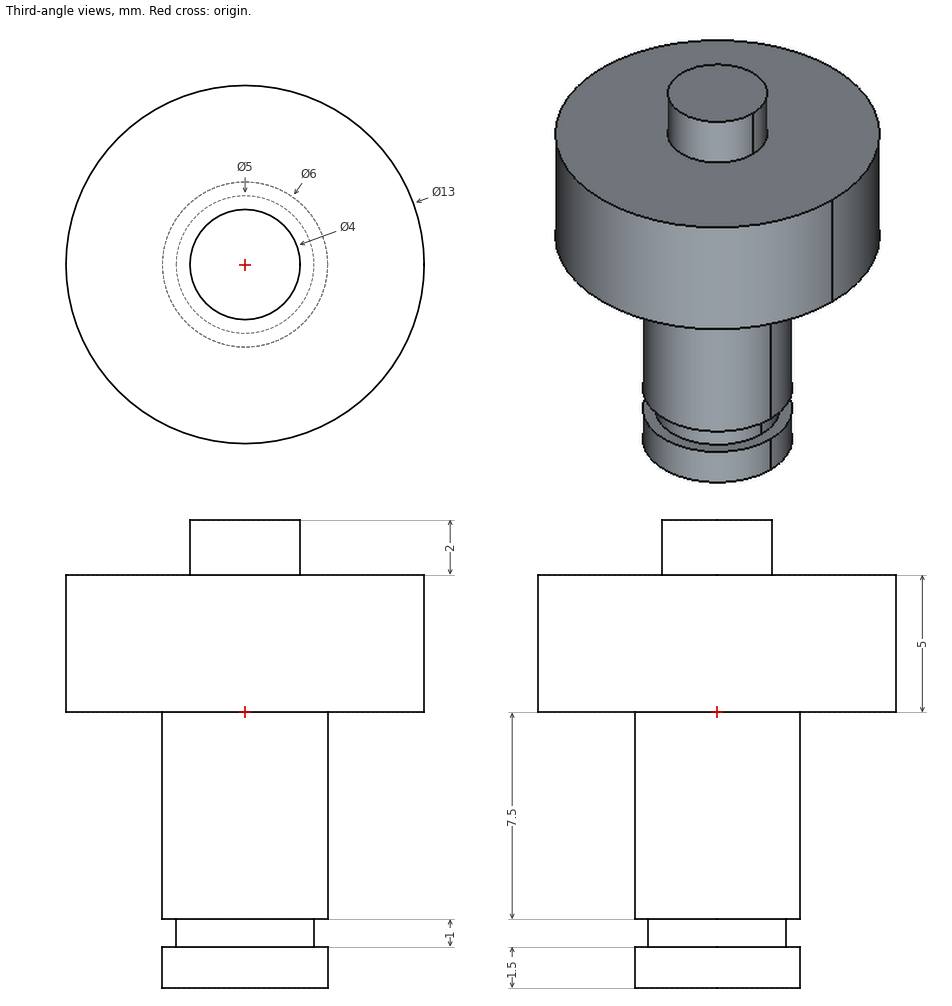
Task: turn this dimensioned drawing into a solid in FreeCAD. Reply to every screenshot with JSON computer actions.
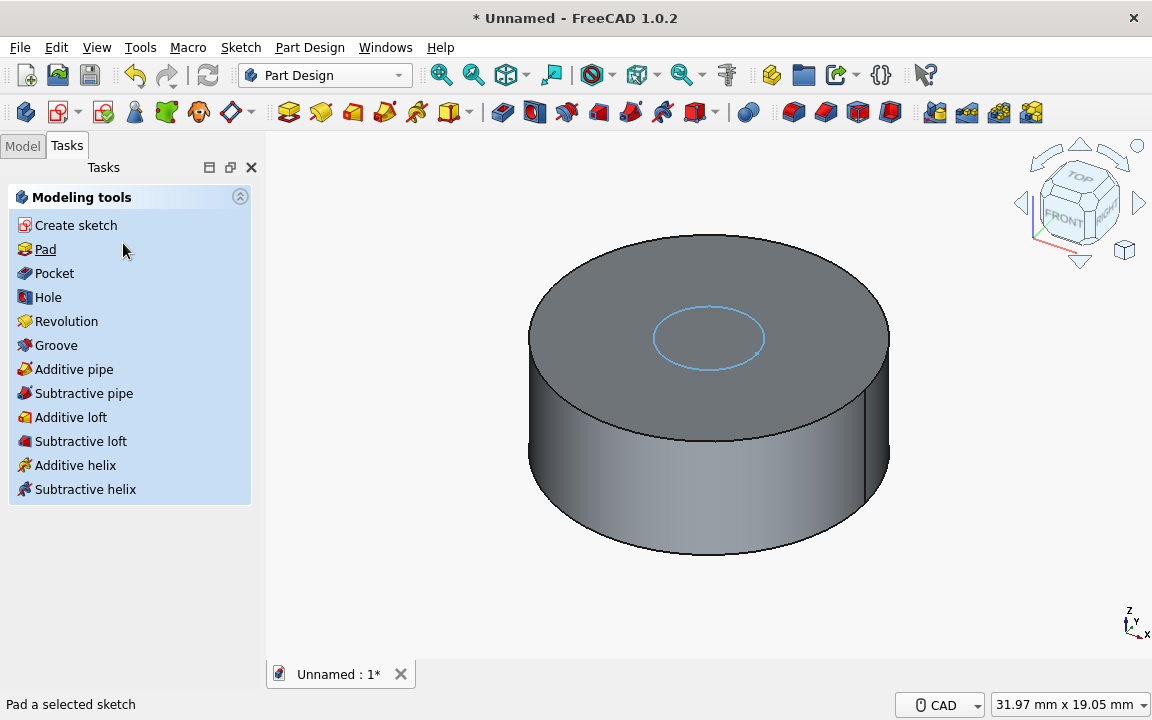
{"action": "left_click", "coordinate": [290, 112]}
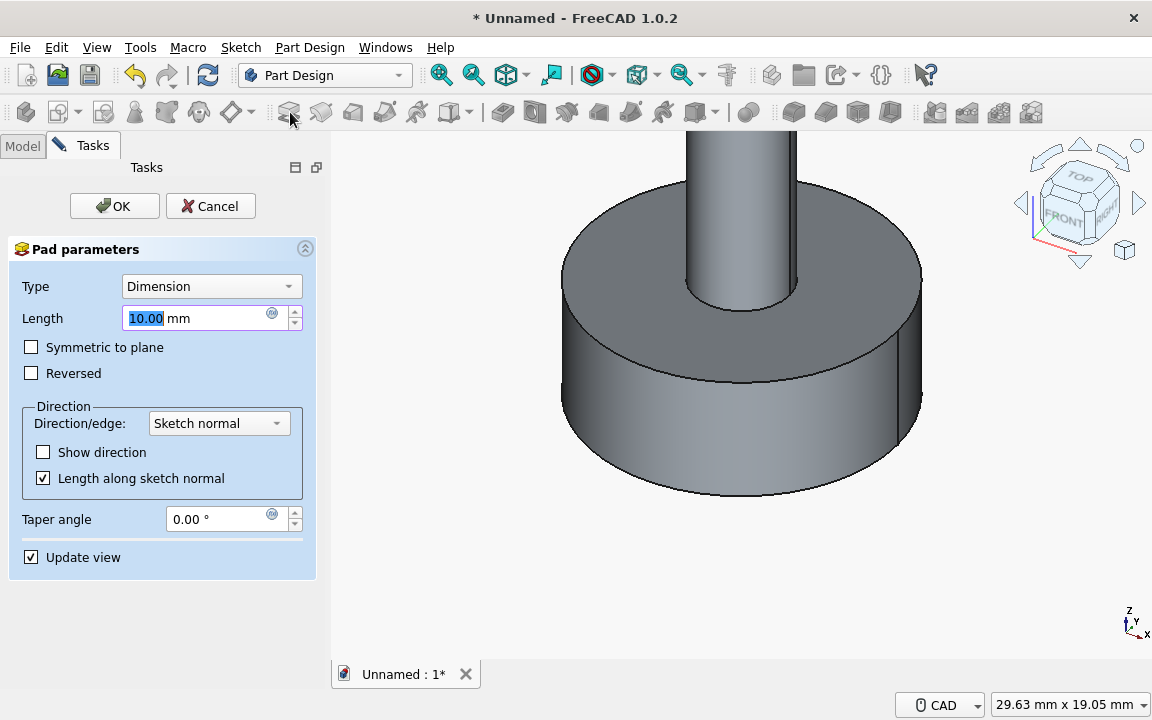
{"action": "type", "text": "2"}
{"action": "key", "text": "Tab"}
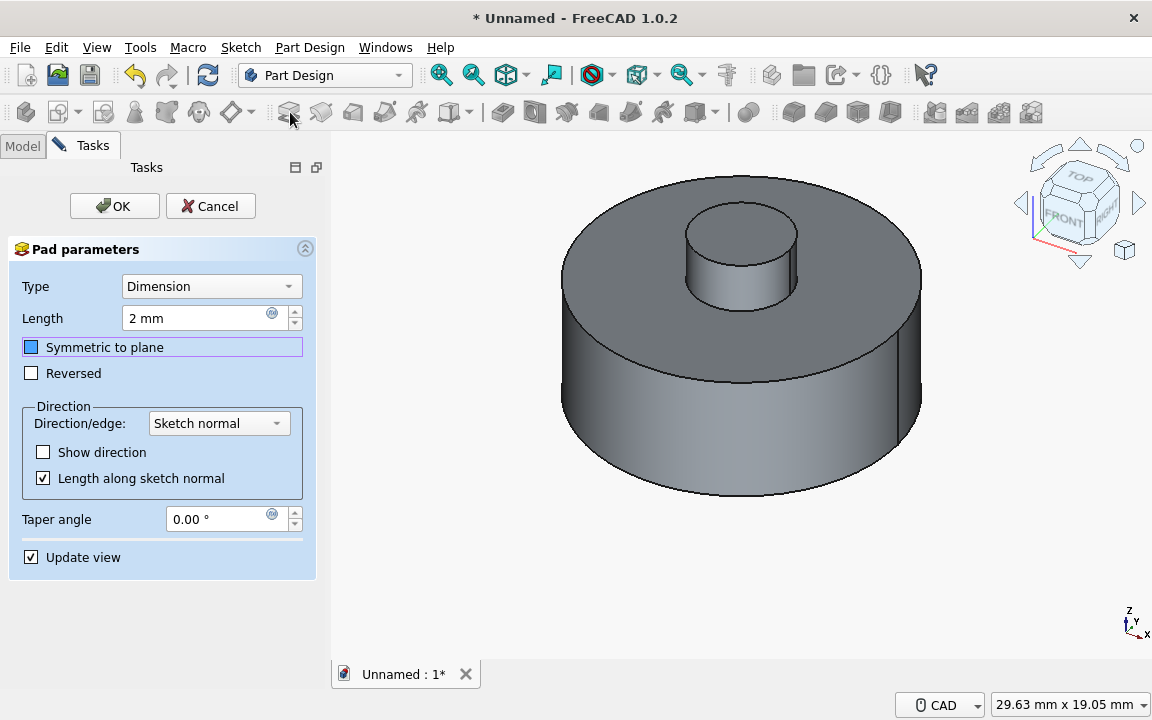
{"action": "left_click", "coordinate": [115, 206]}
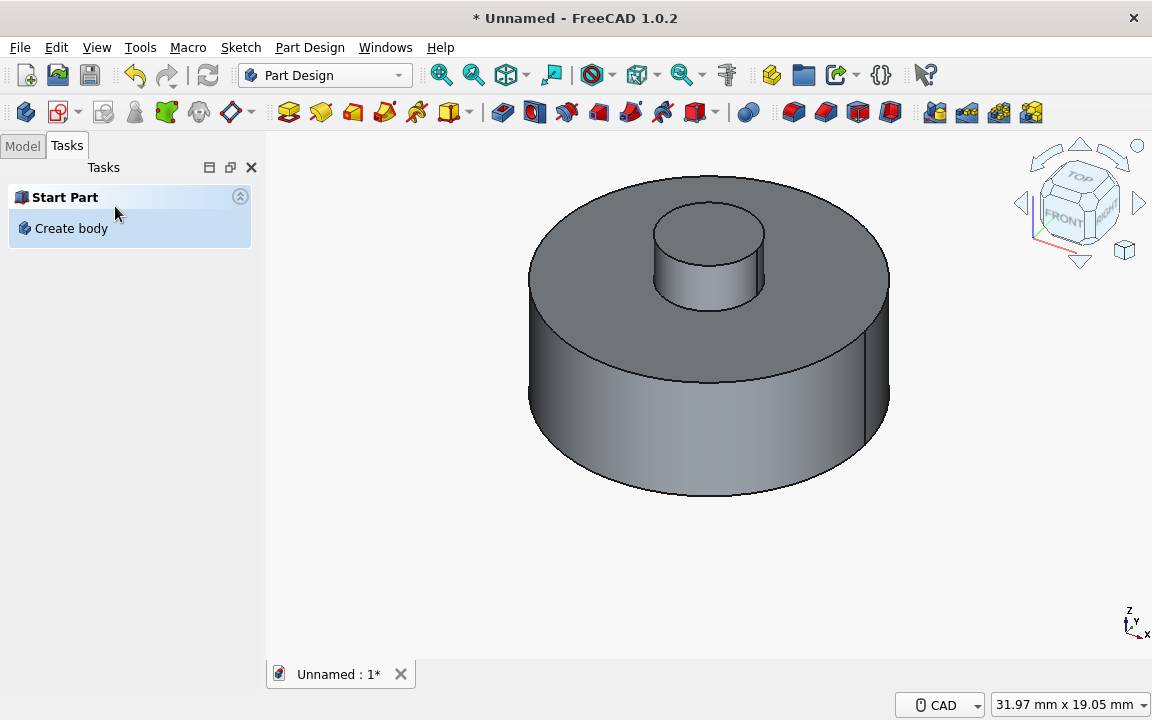
{"action": "key", "text": "v f"}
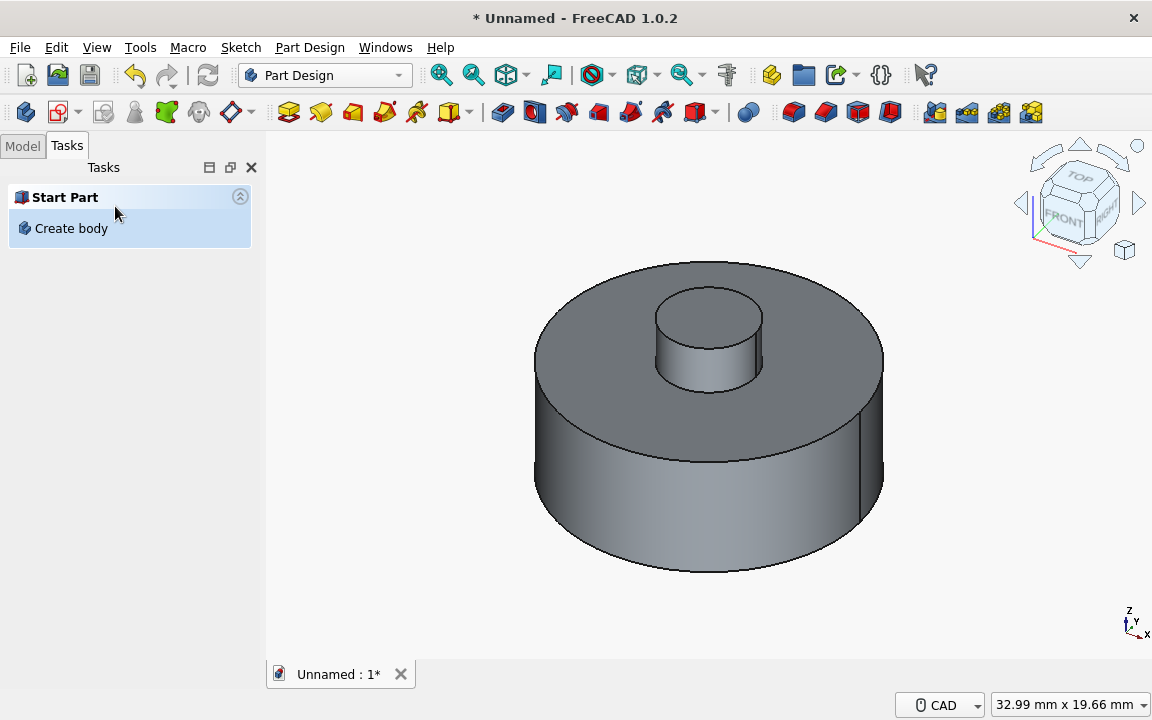
{"action": "key", "text": "5"}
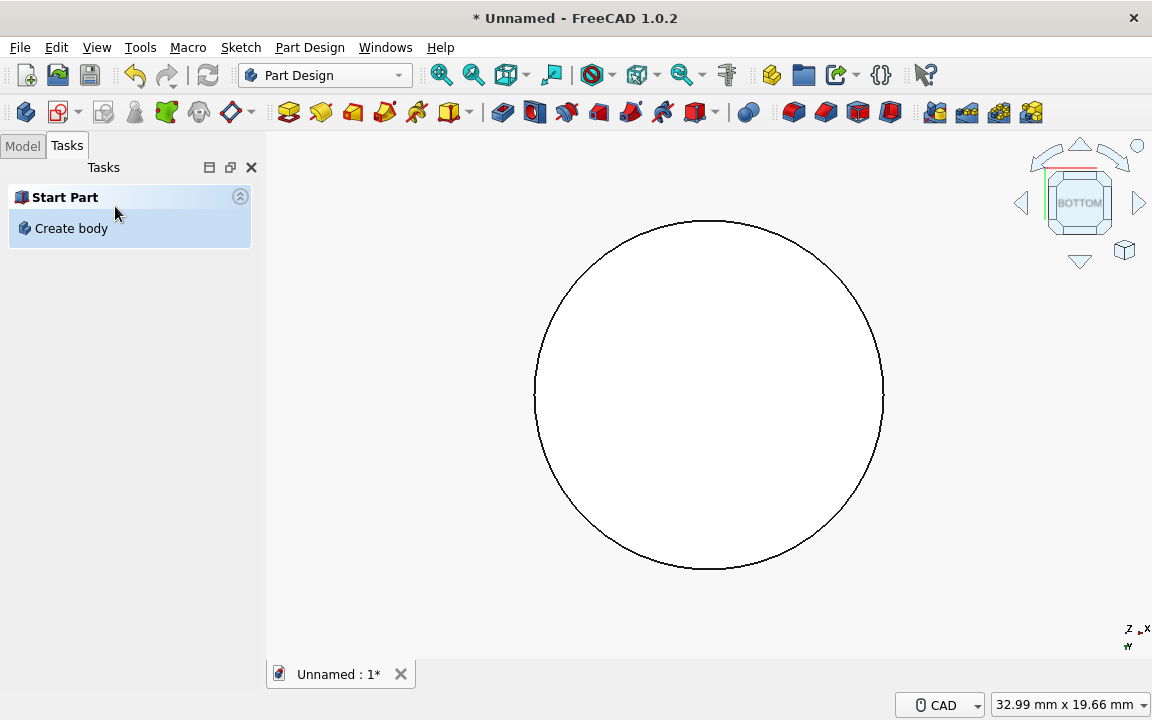
{"action": "left_click", "coordinate": [709, 394]}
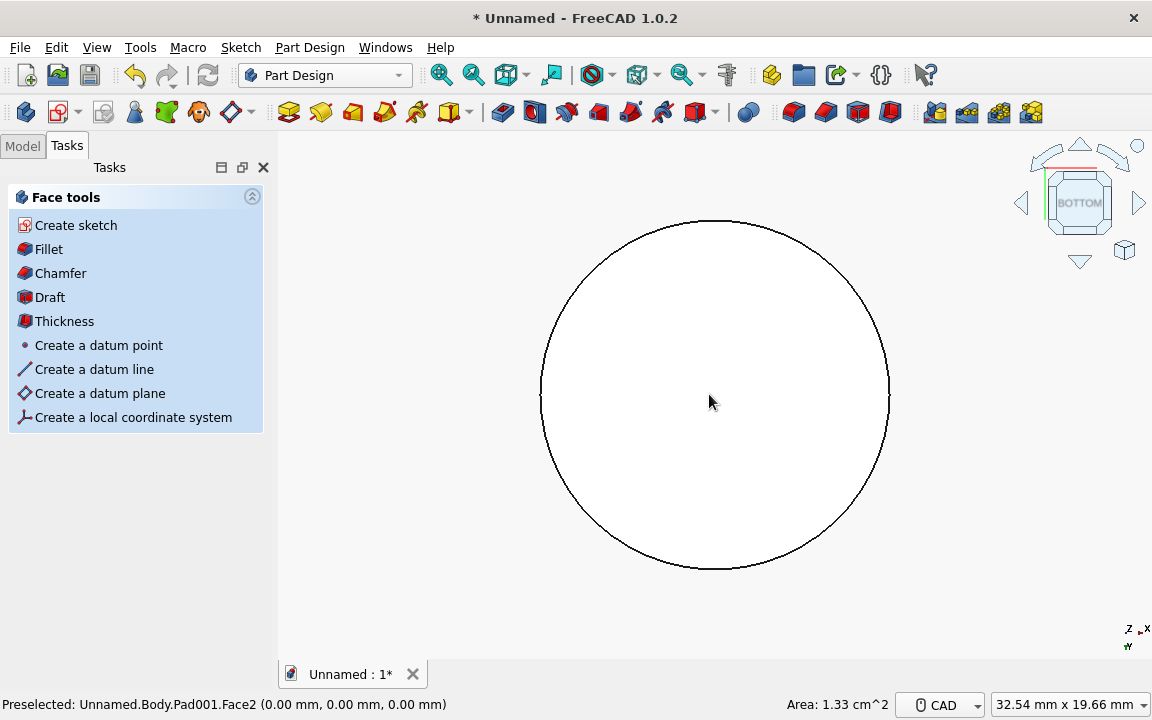
{"action": "left_click", "coordinate": [58, 112]}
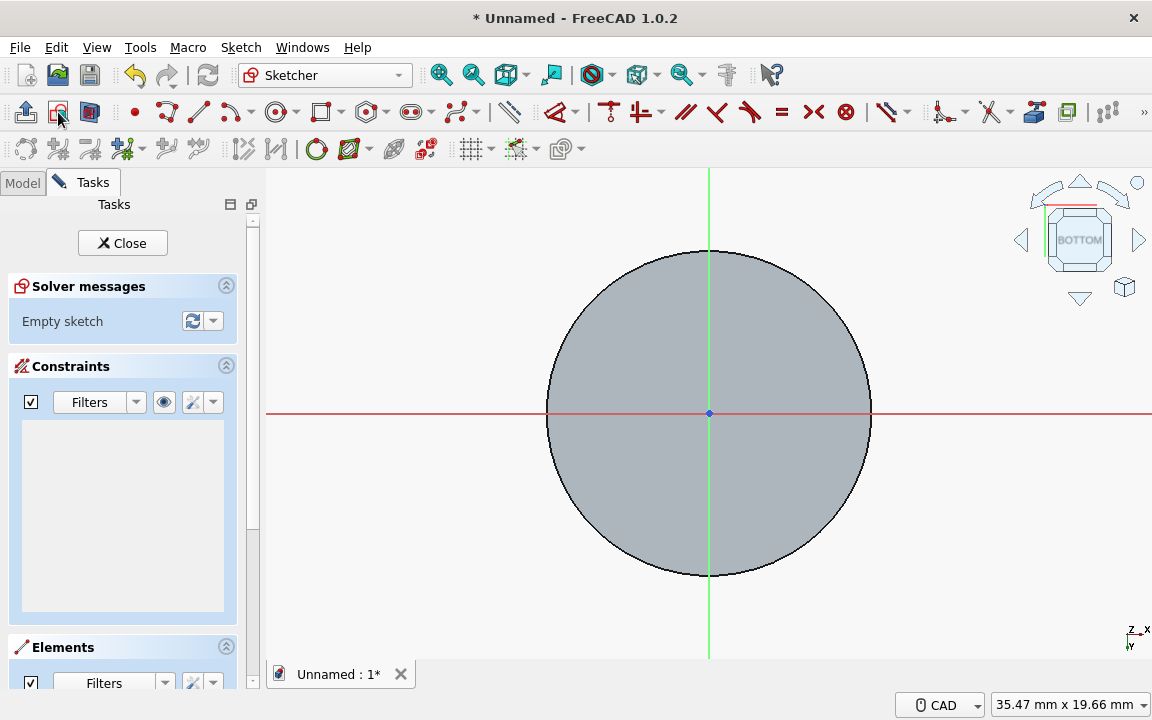
{"action": "scroll", "coordinate": [765, 413], "scroll_direction": "up", "scroll_amount": 4}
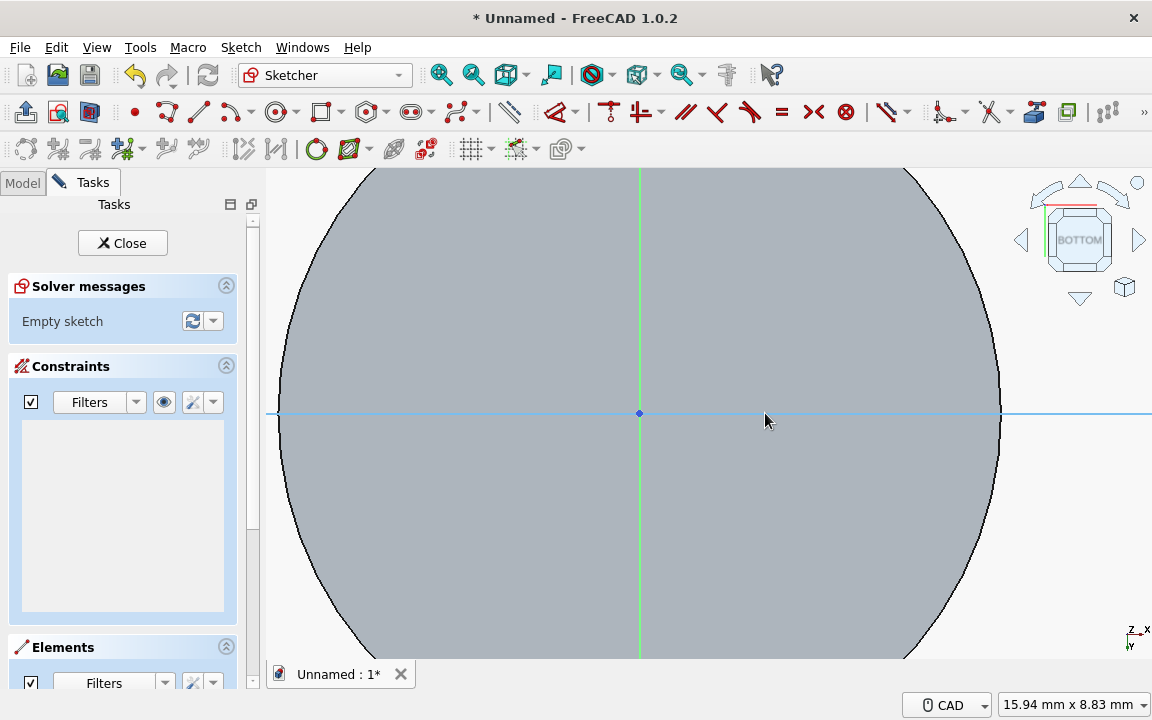
{"action": "key", "text": "g c"}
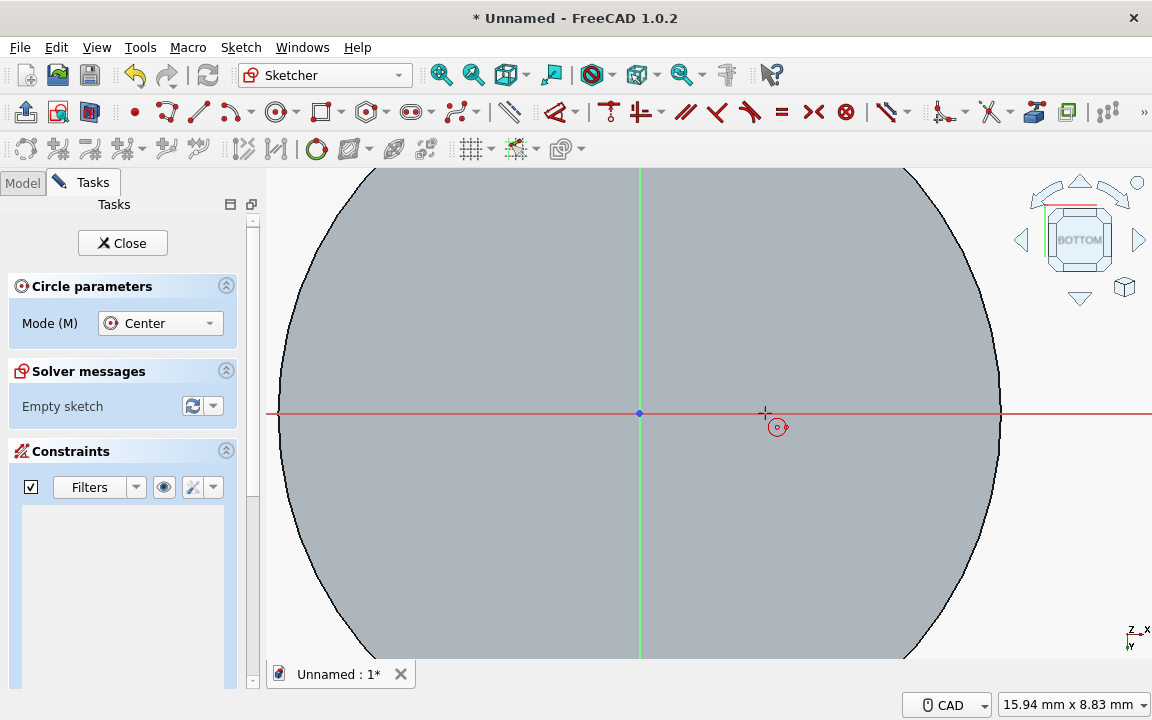
{"action": "left_click", "coordinate": [640, 414]}
{"action": "left_click", "coordinate": [758, 296]}
{"action": "key", "text": "Escape"}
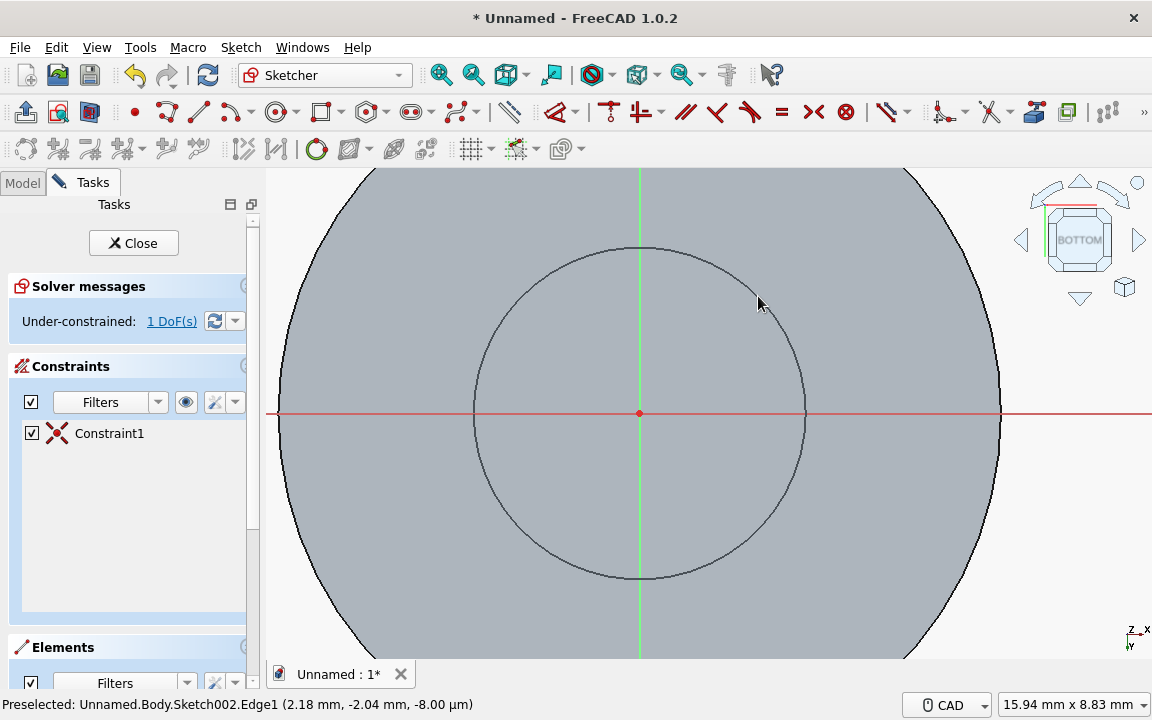
{"action": "key", "text": "d"}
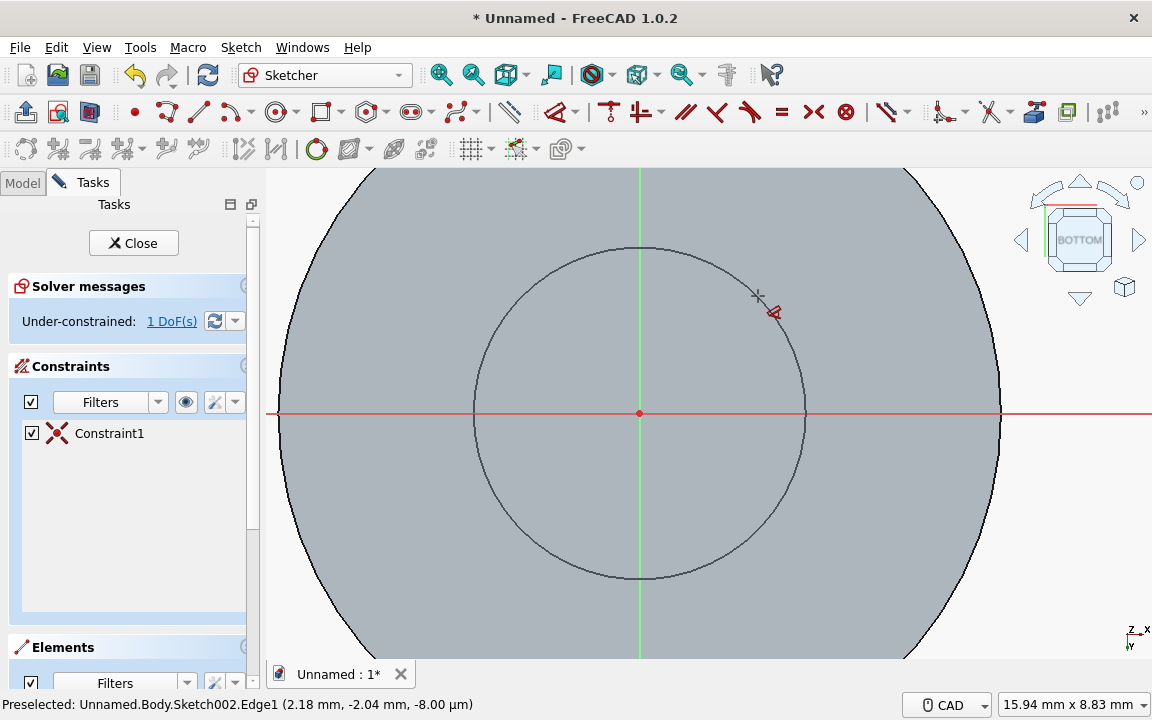
{"action": "left_click", "coordinate": [757, 296]}
{"action": "left_click", "coordinate": [780, 273]}